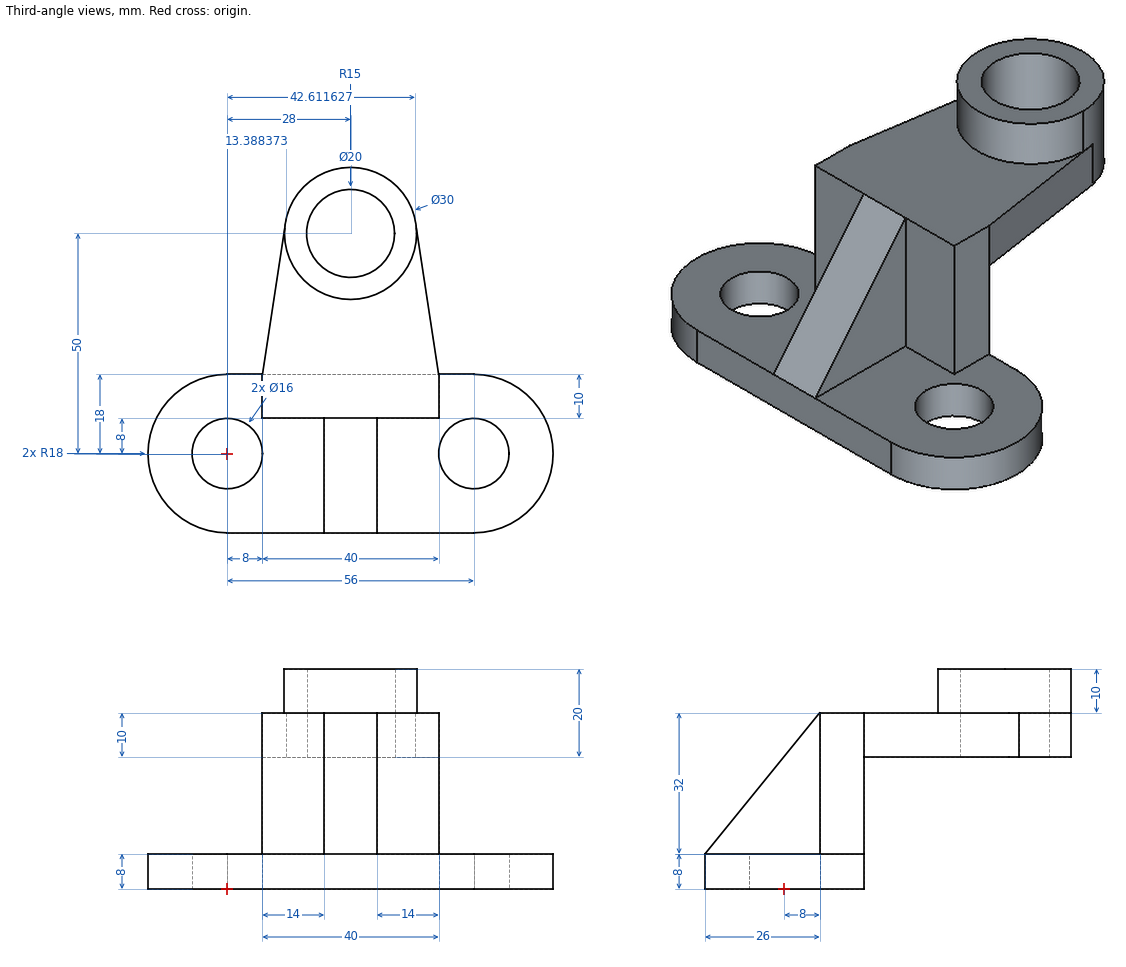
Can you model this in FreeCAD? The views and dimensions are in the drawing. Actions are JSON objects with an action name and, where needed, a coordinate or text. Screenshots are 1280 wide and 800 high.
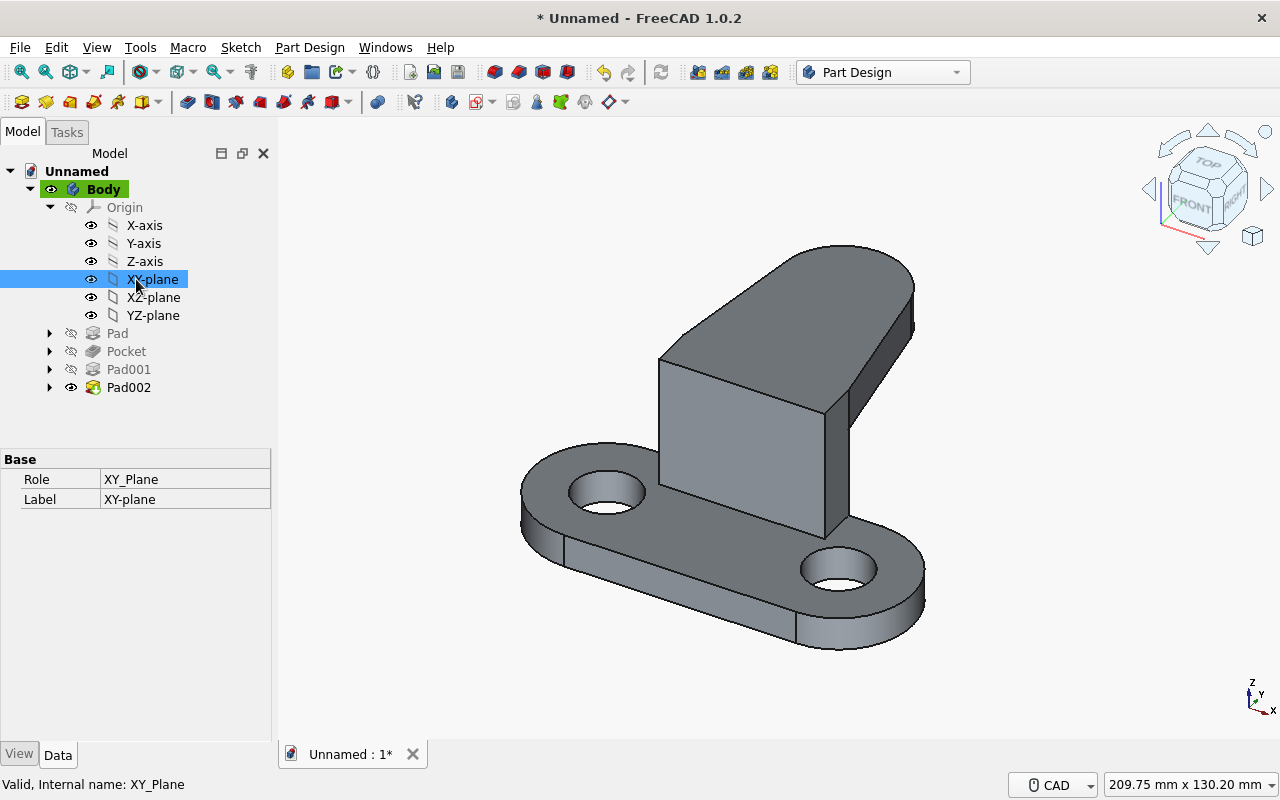
{"action": "left_click", "coordinate": [610, 102]}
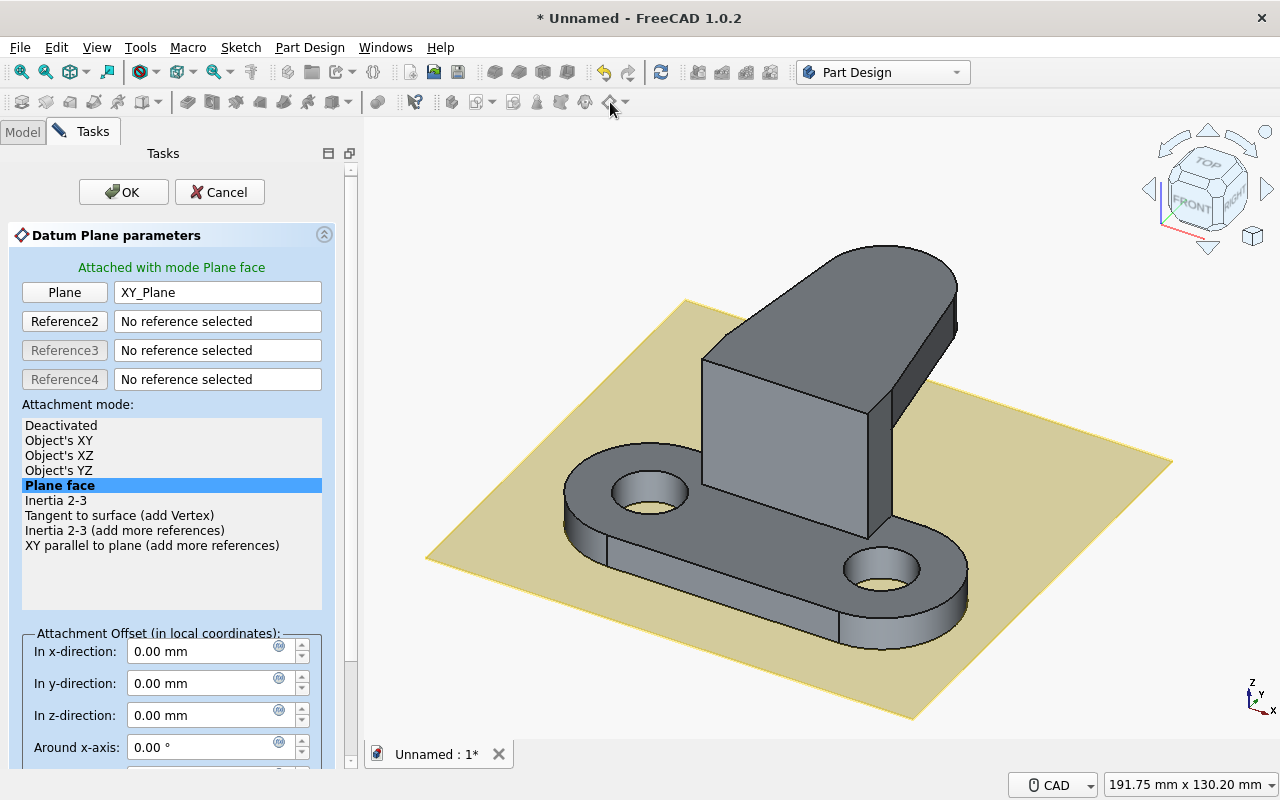
{"action": "triple_click", "coordinate": [210, 715]}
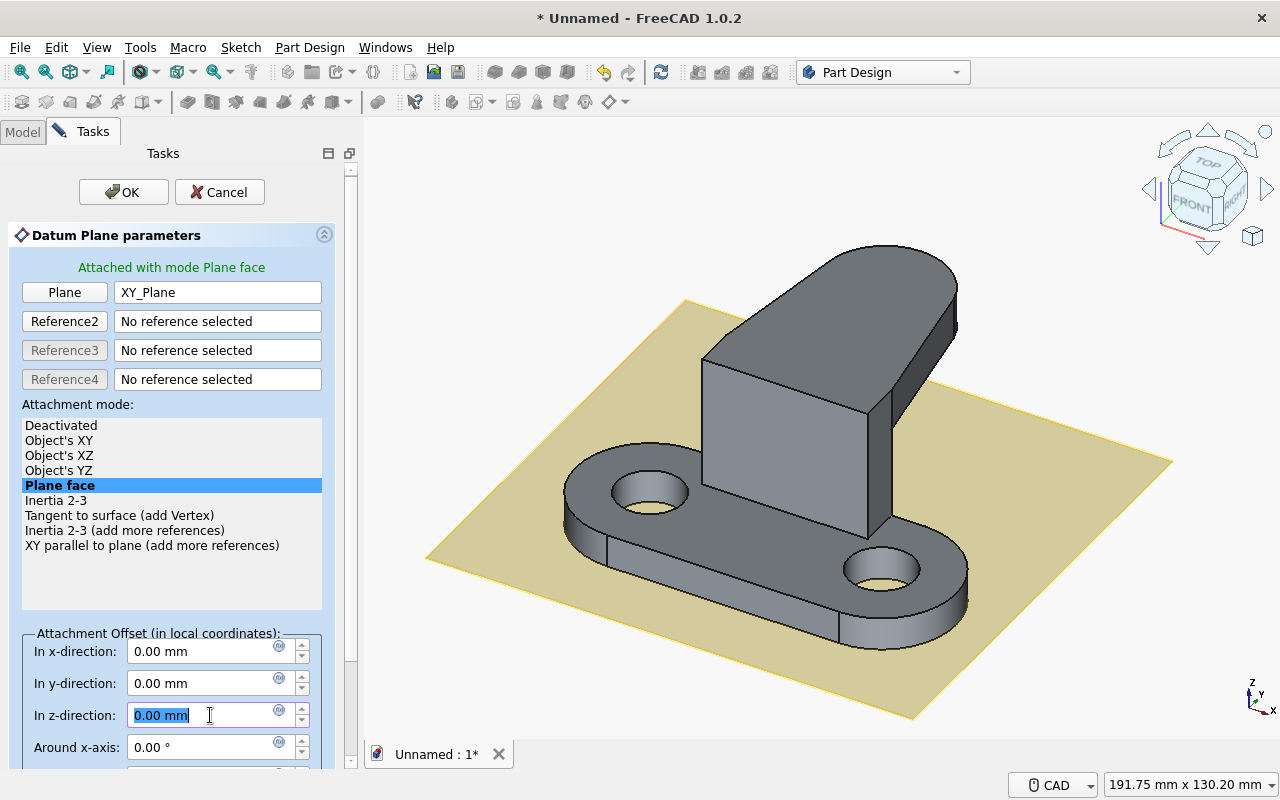
{"action": "type", "text": "50"}
{"action": "key", "text": "Tab"}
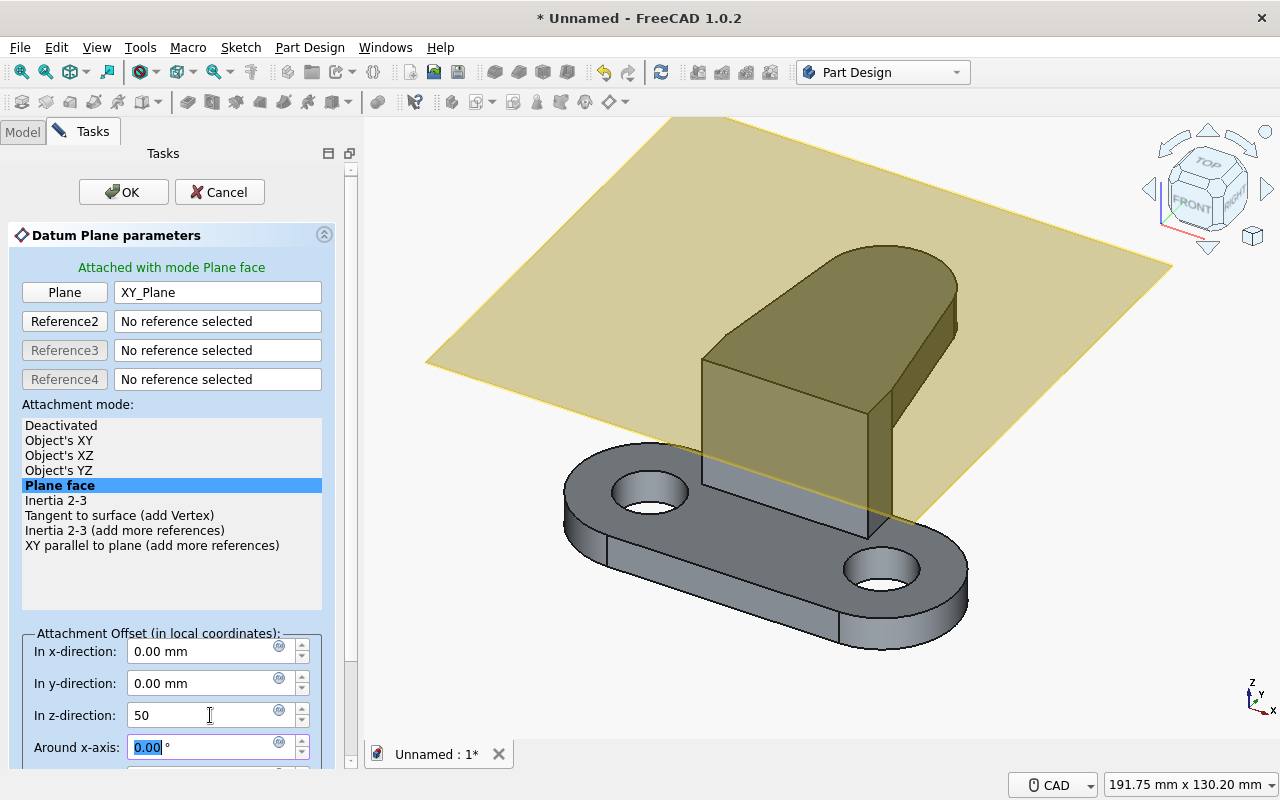
{"action": "left_click", "coordinate": [124, 192]}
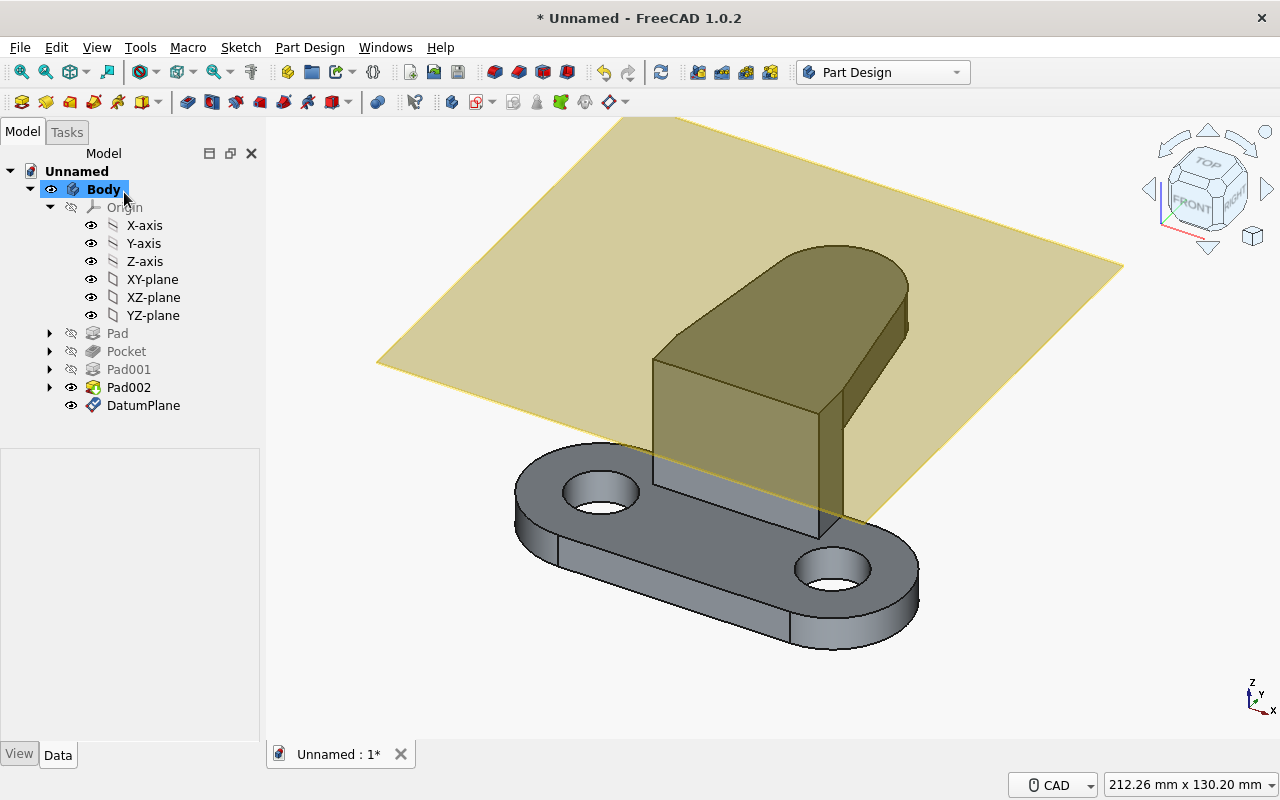
{"action": "left_click", "coordinate": [116, 405]}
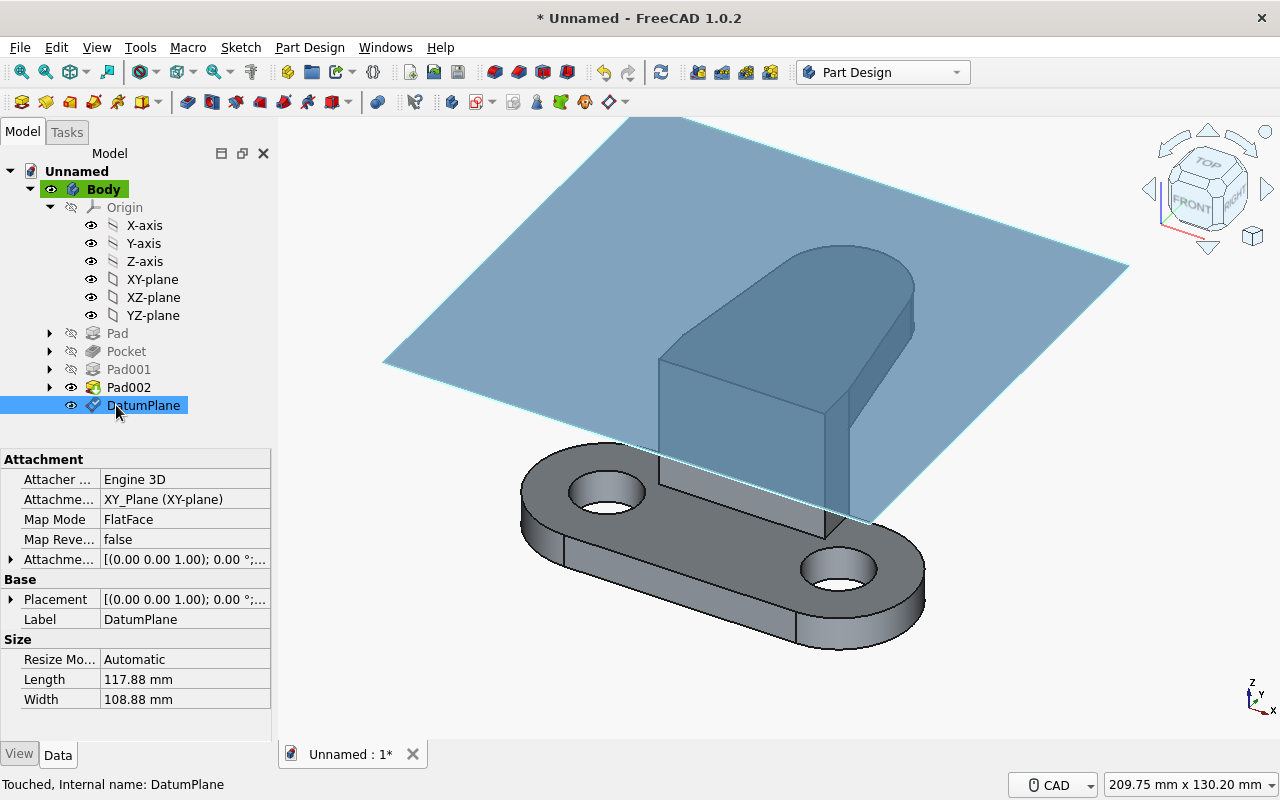
{"action": "left_click", "coordinate": [476, 102]}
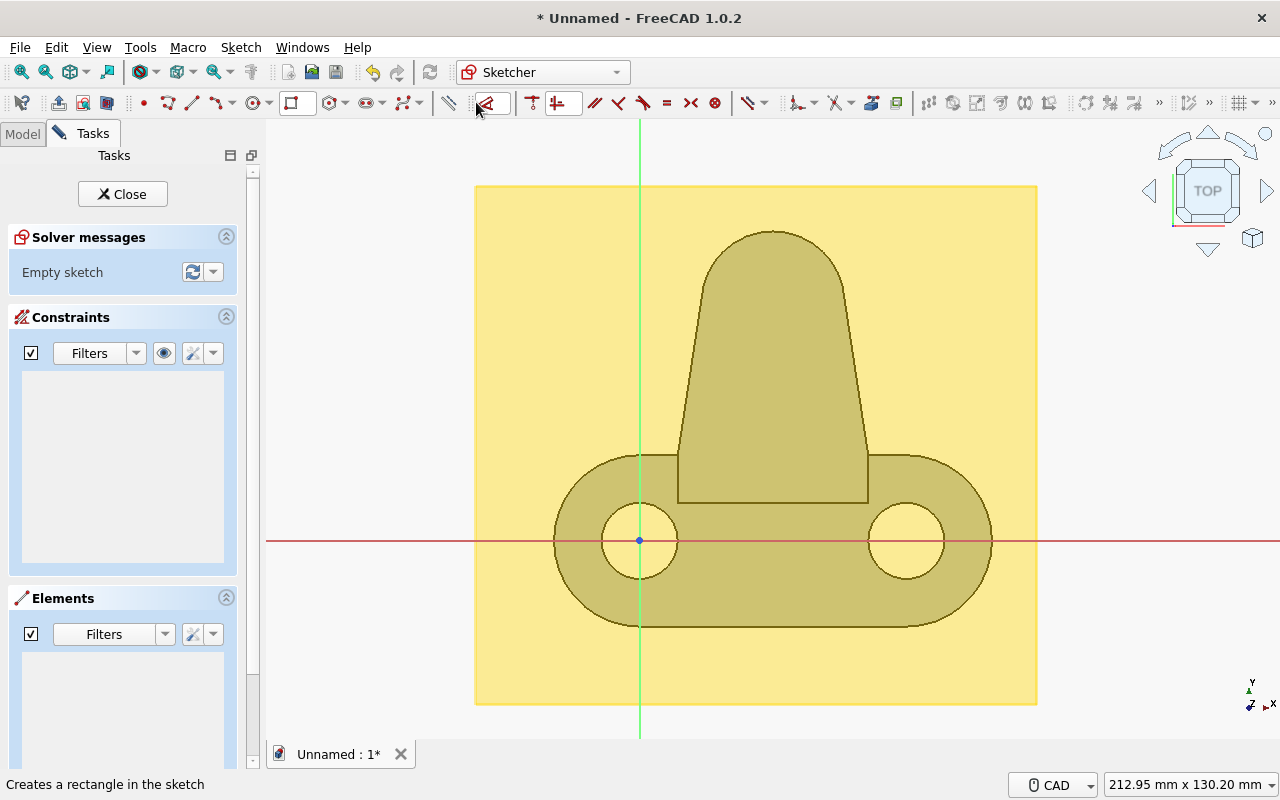
{"action": "left_click", "coordinate": [254, 104]}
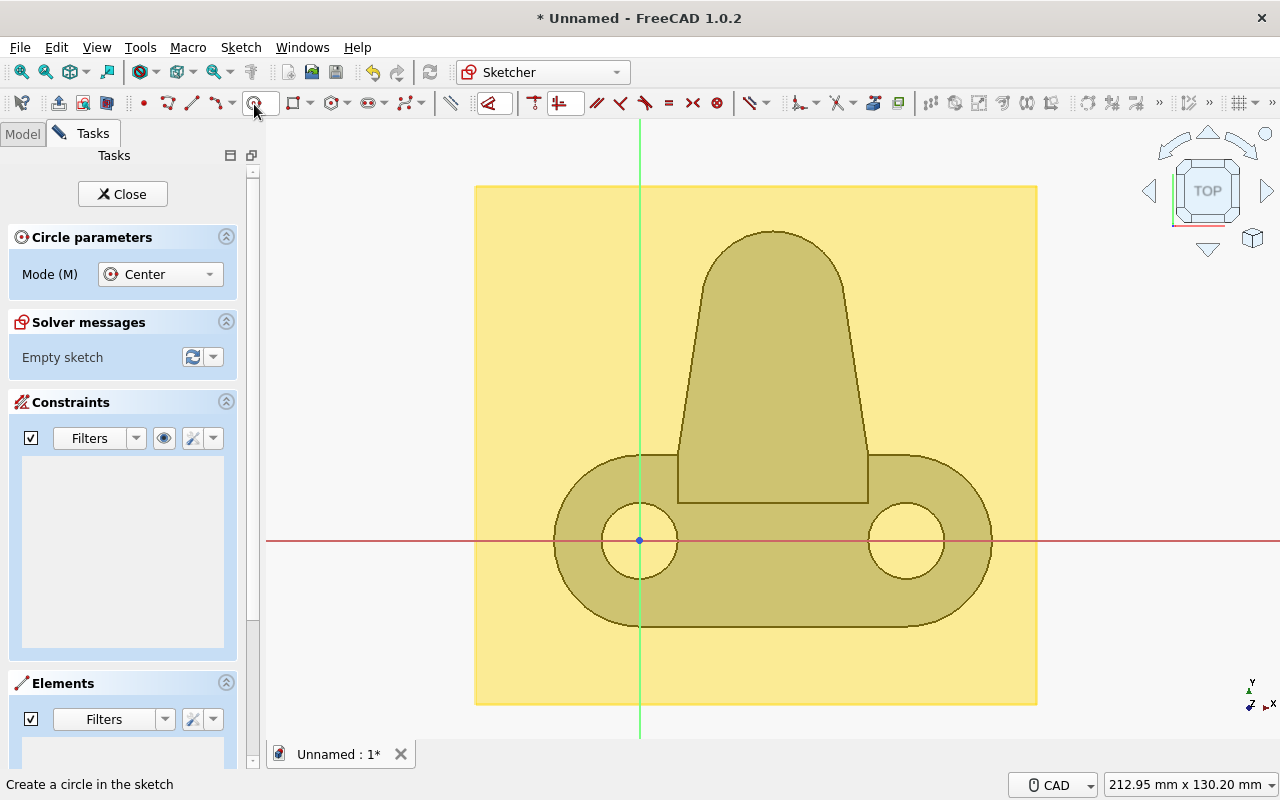
{"action": "left_click", "coordinate": [773, 303]}
{"action": "mouse_move", "coordinate": [824, 252]}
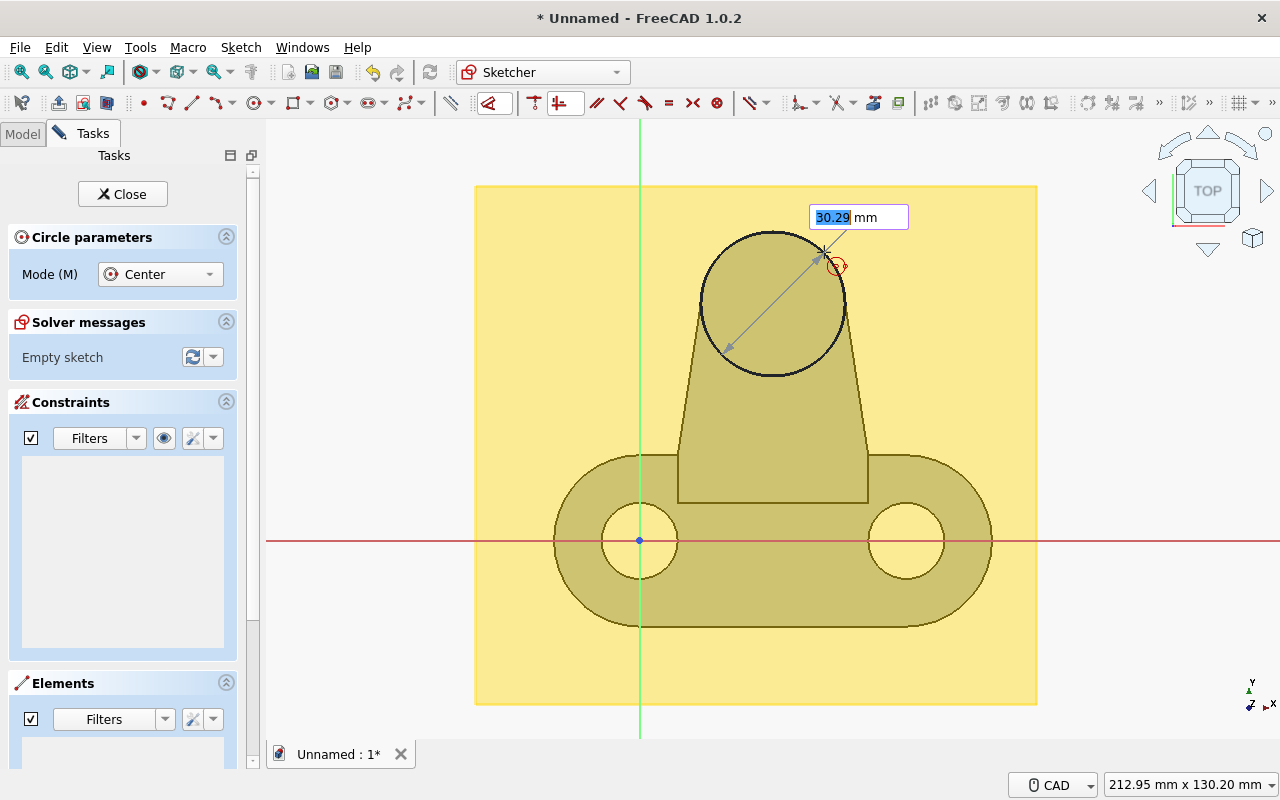
{"action": "type", "text": "30"}
{"action": "key", "text": "Return"}
{"action": "key", "text": "Escape"}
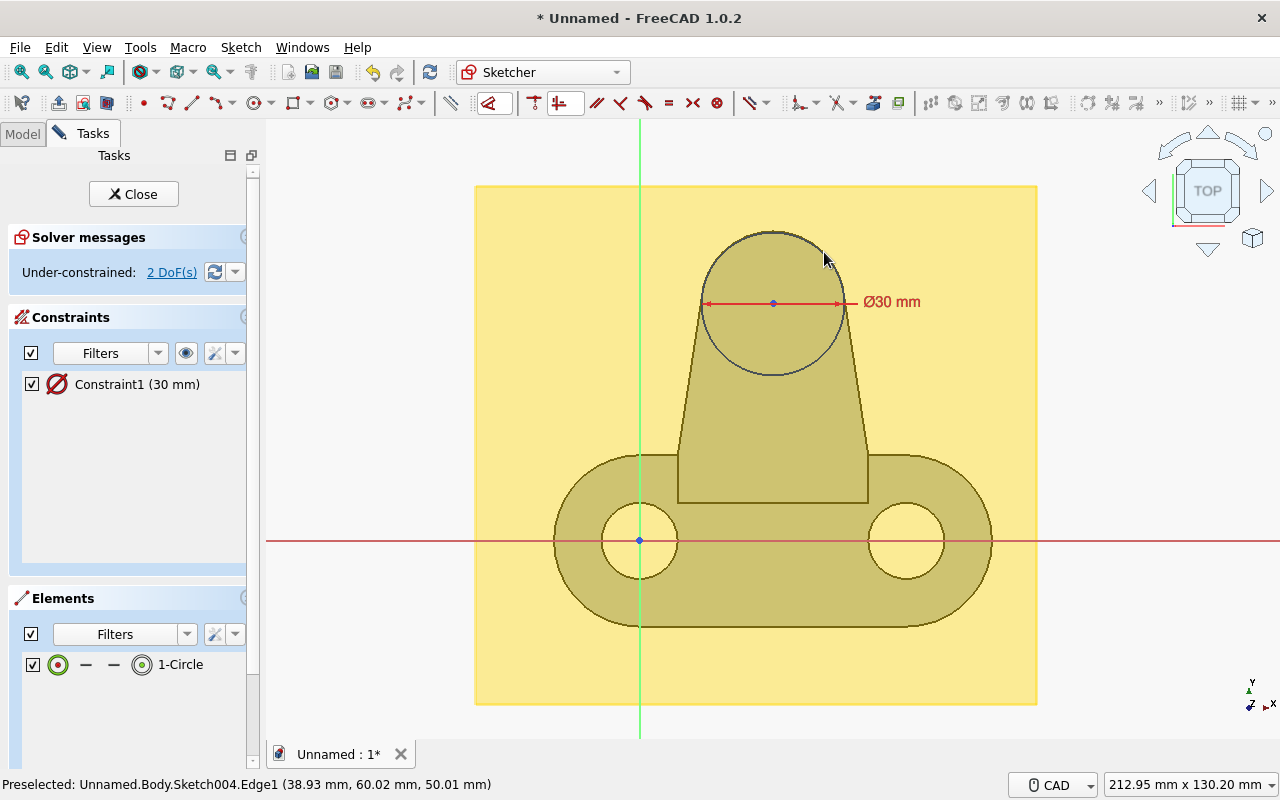
{"action": "left_click", "coordinate": [773, 304]}